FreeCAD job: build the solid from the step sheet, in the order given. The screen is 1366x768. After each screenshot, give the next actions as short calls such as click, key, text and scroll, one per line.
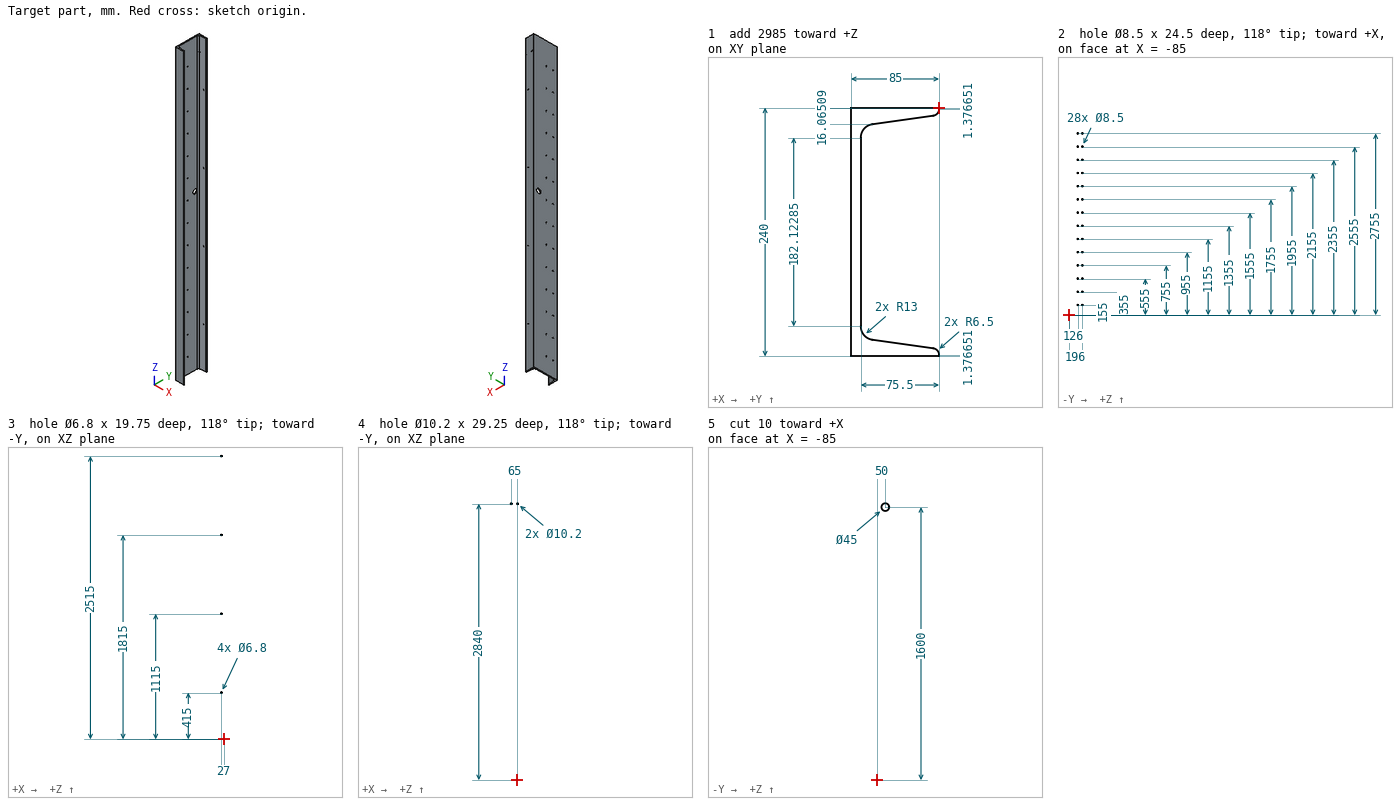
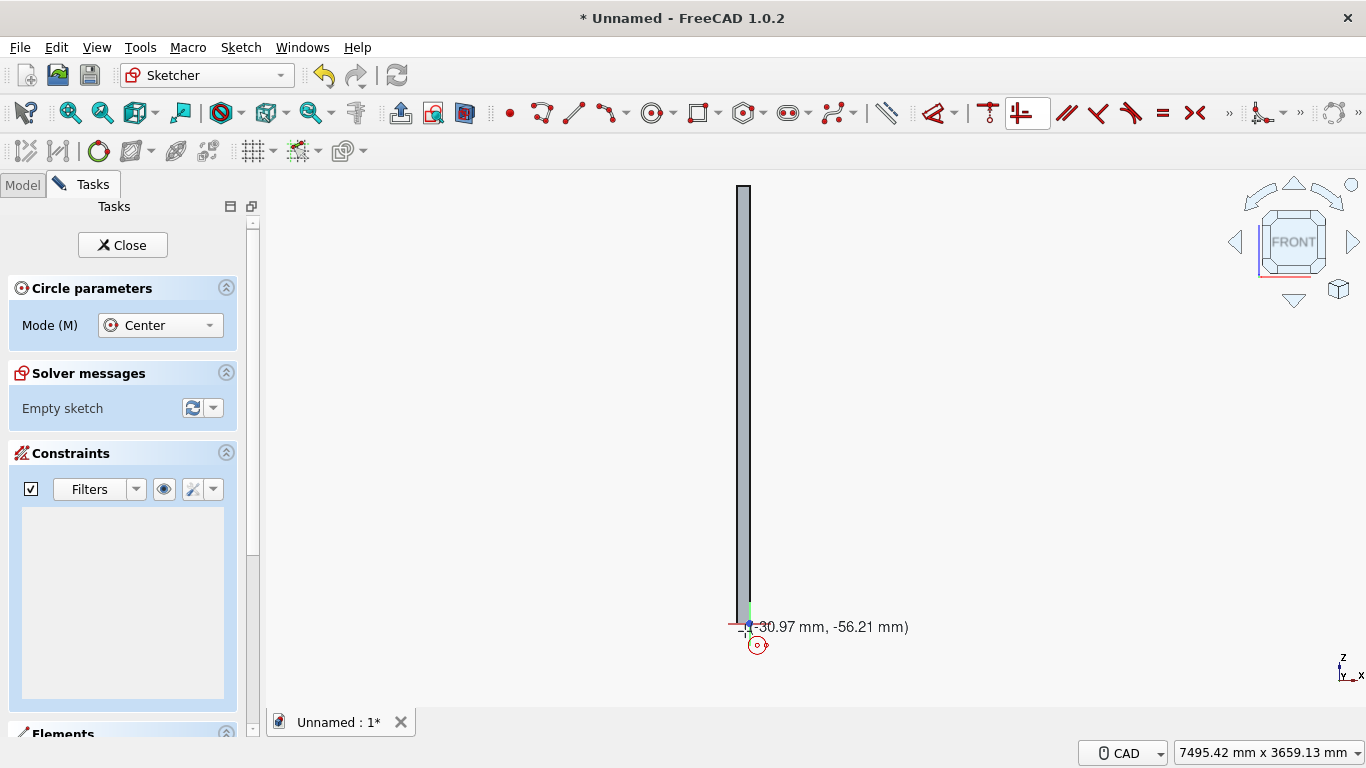
scroll(746, 563, up, 7)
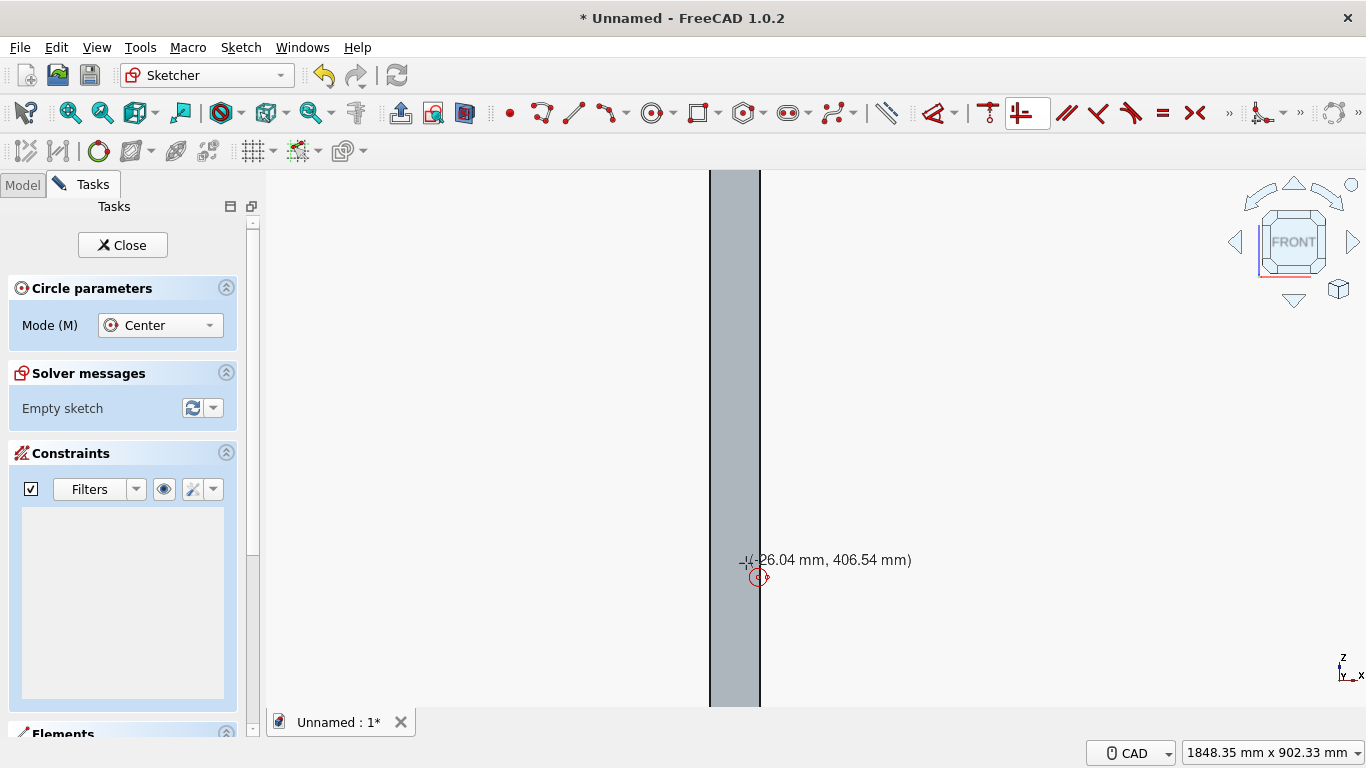
click(744, 560)
move(746, 558)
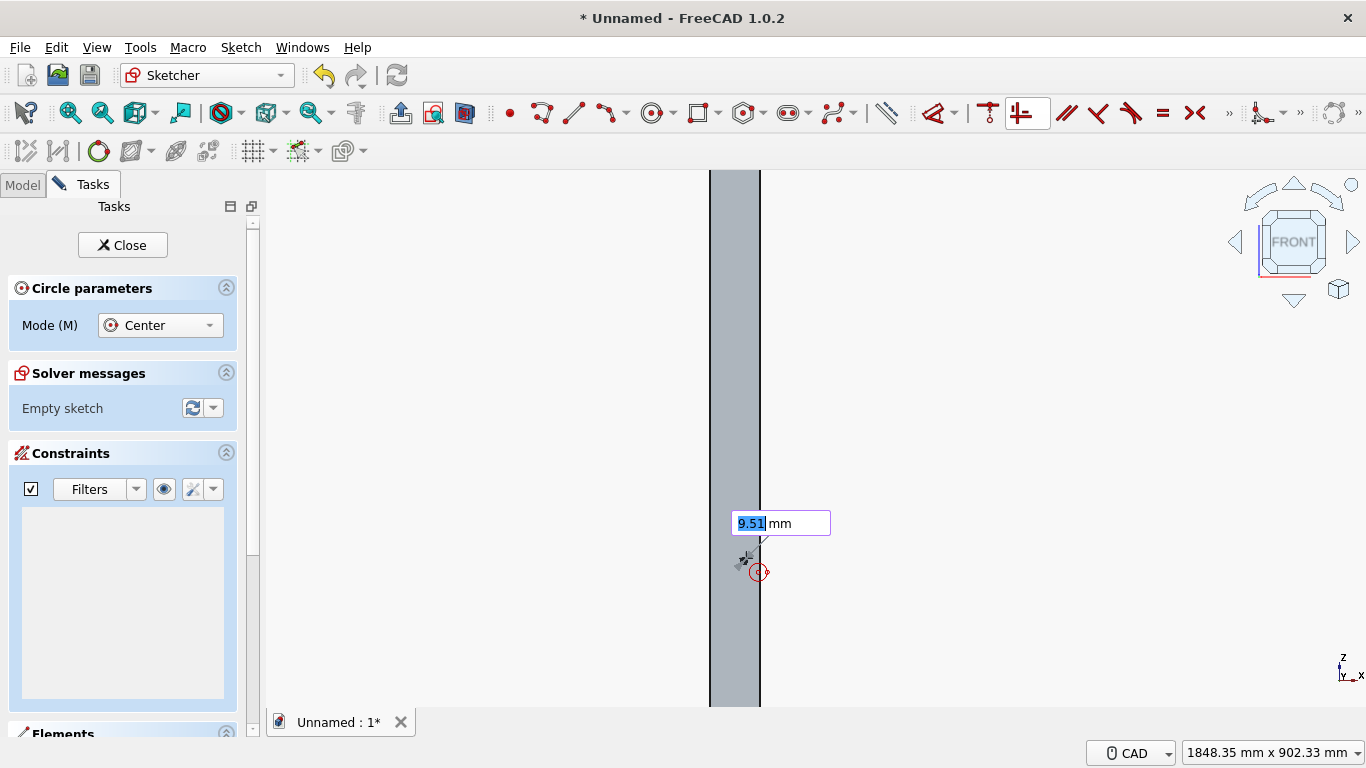
text(6.8)
key(Return)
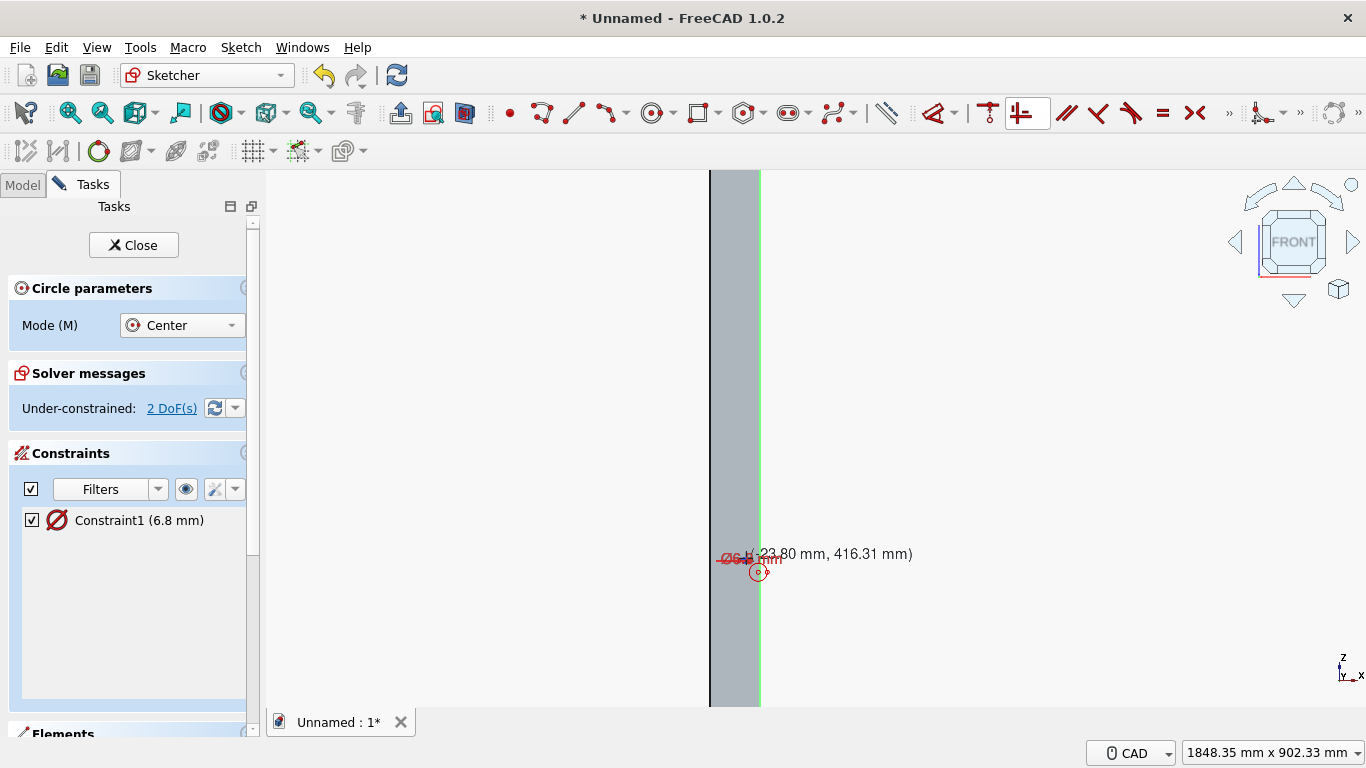
scroll(746, 563, down, 7)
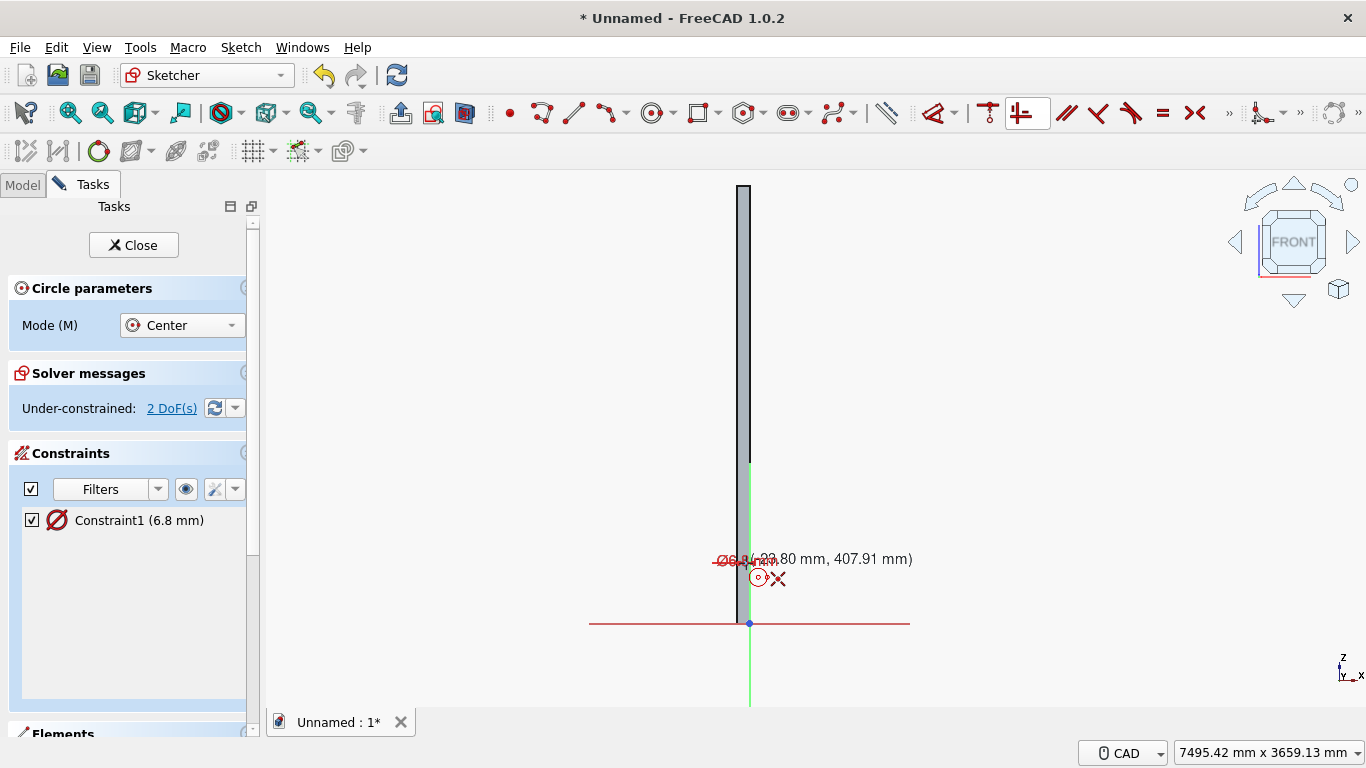
scroll(746, 460, up, 20)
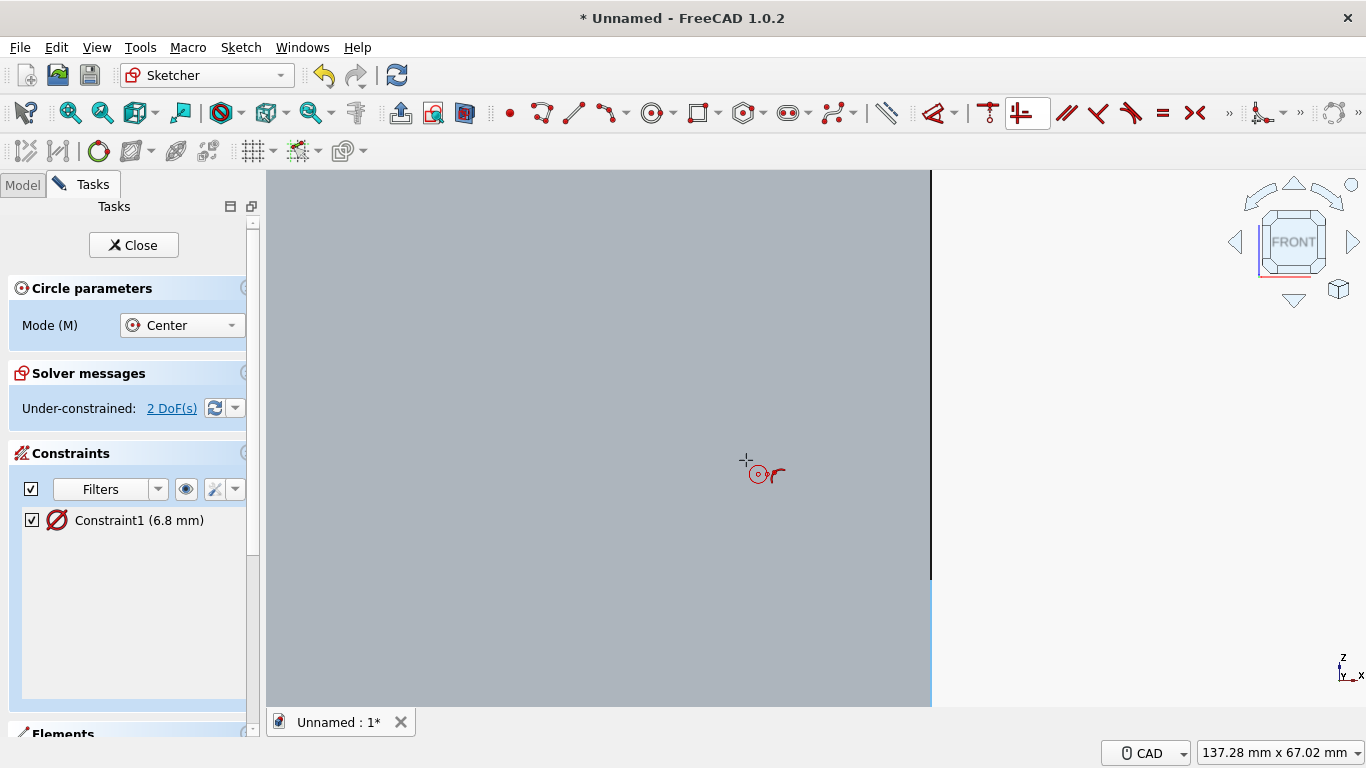
scroll(748, 438, down, 15)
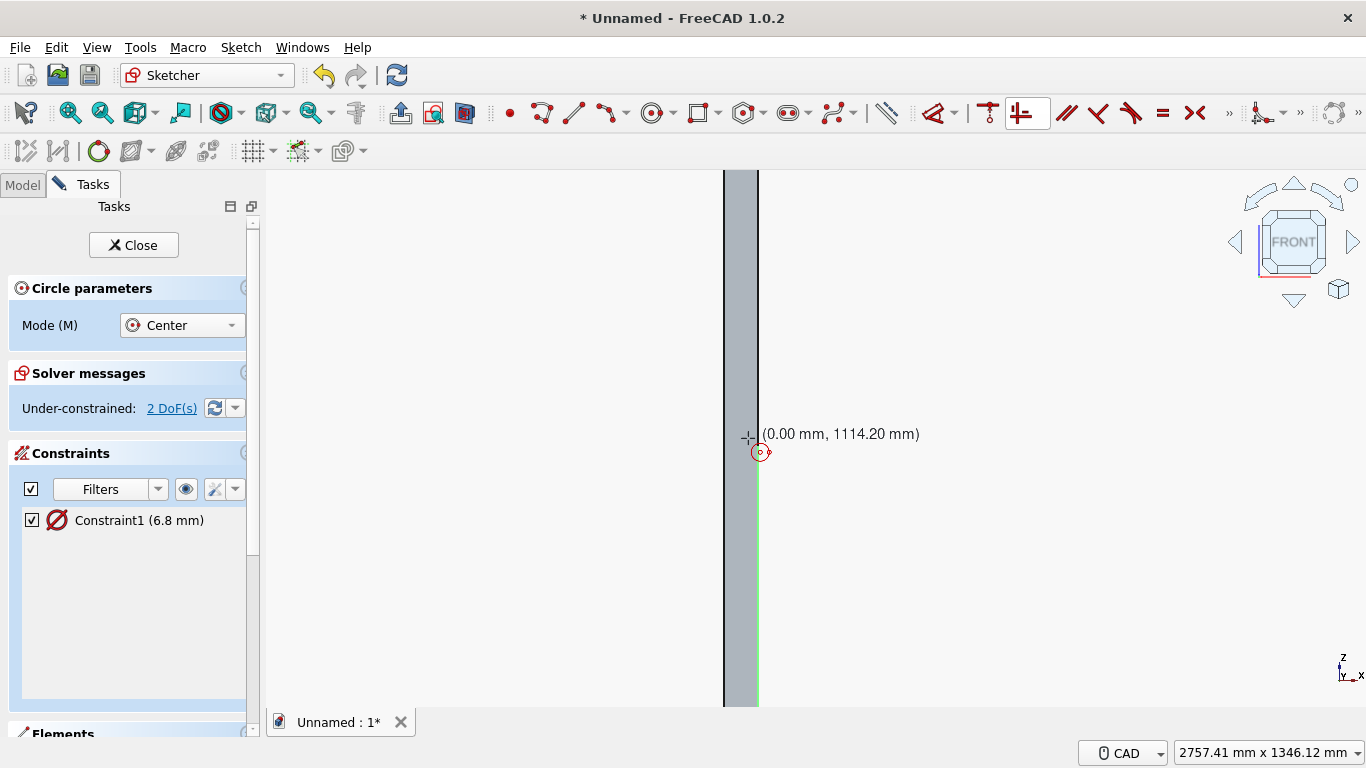
scroll(745, 472, down, 5)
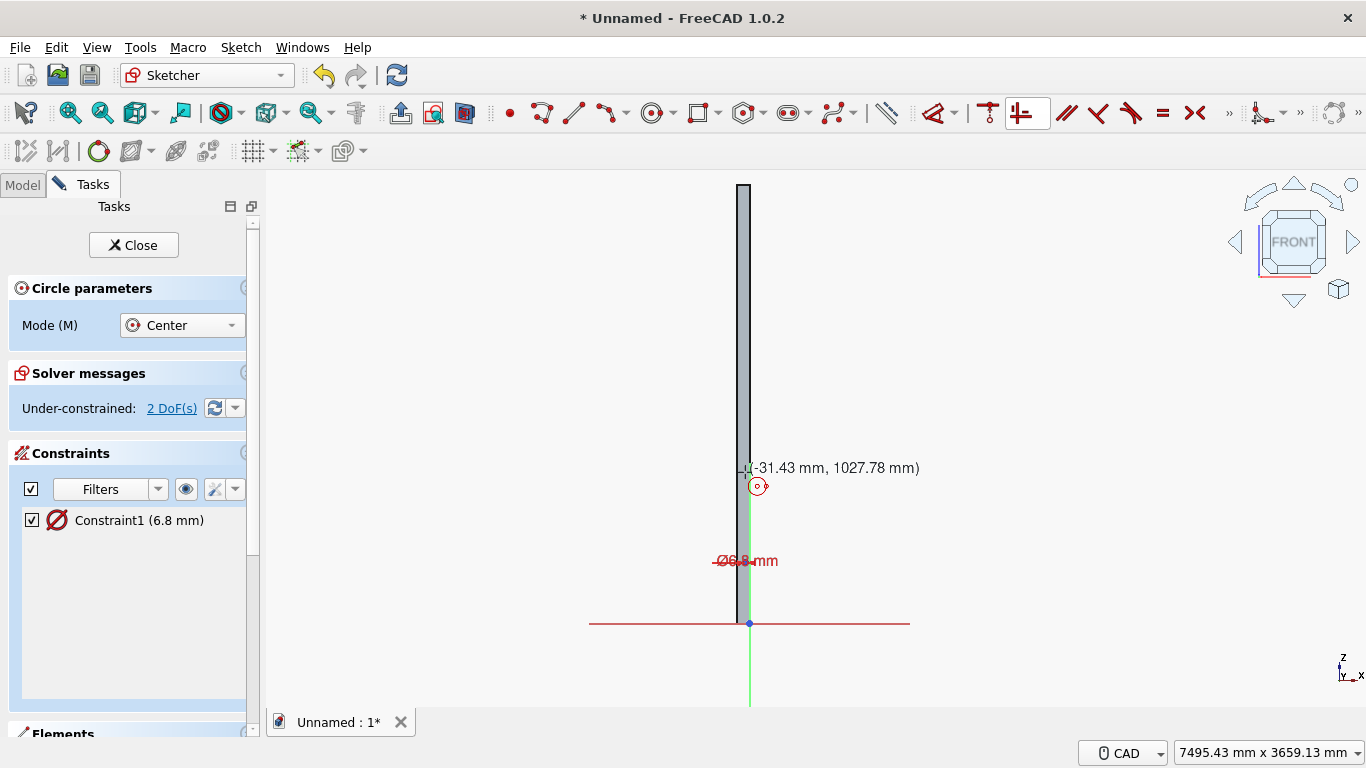
scroll(746, 460, up, 7)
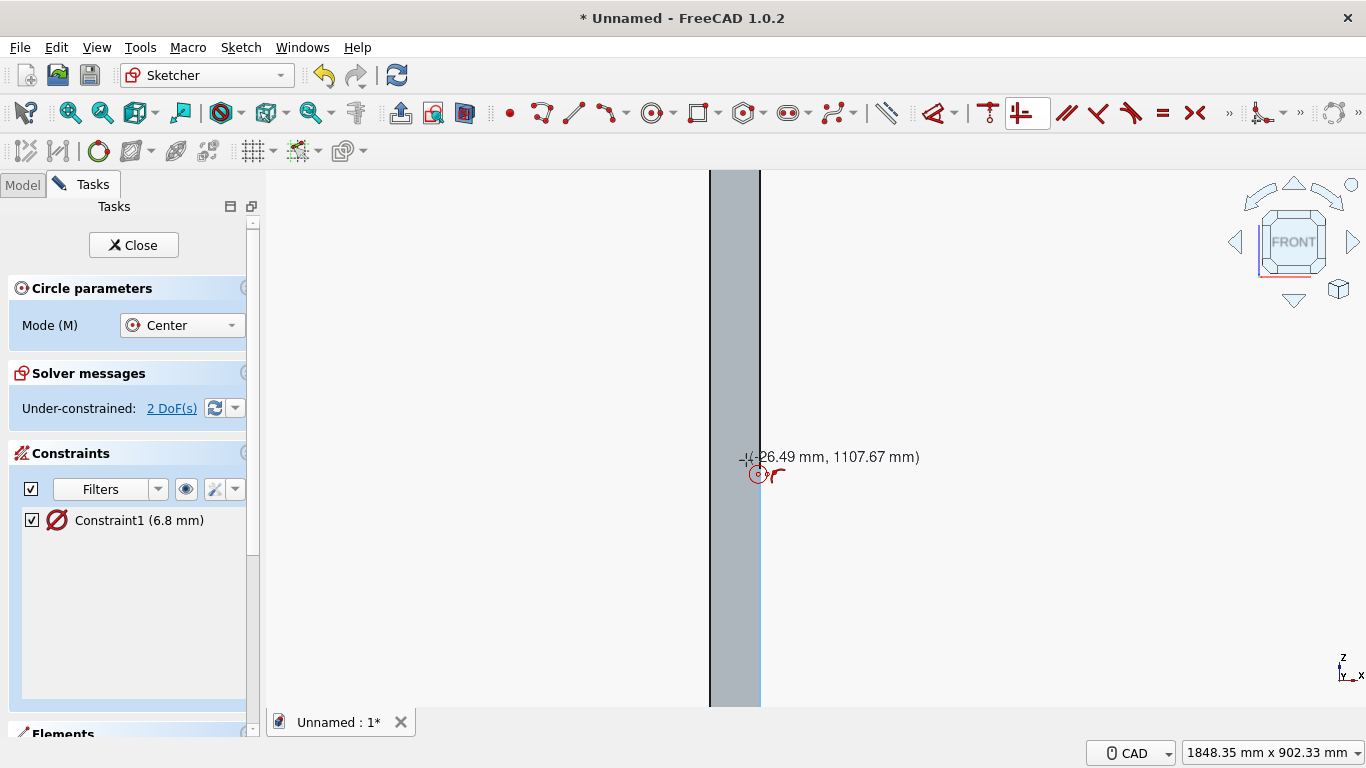
click(744, 458)
move(746, 457)